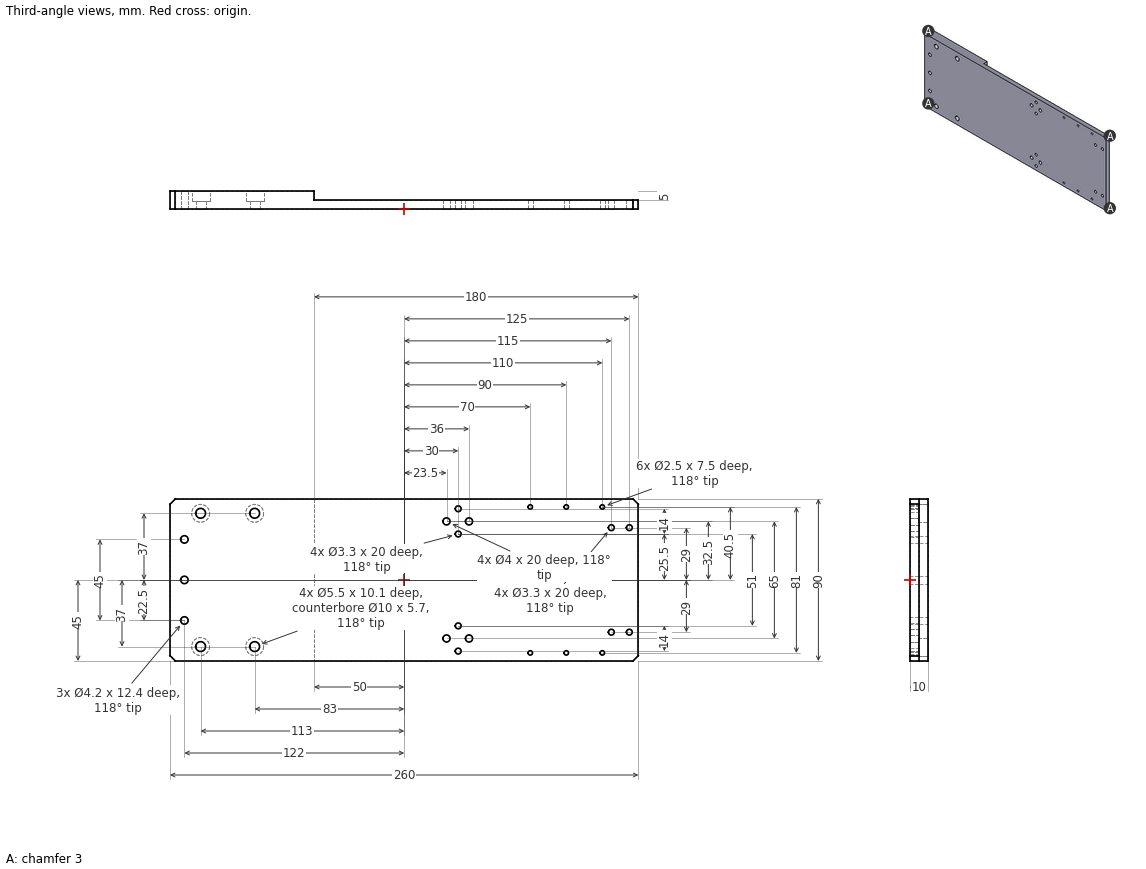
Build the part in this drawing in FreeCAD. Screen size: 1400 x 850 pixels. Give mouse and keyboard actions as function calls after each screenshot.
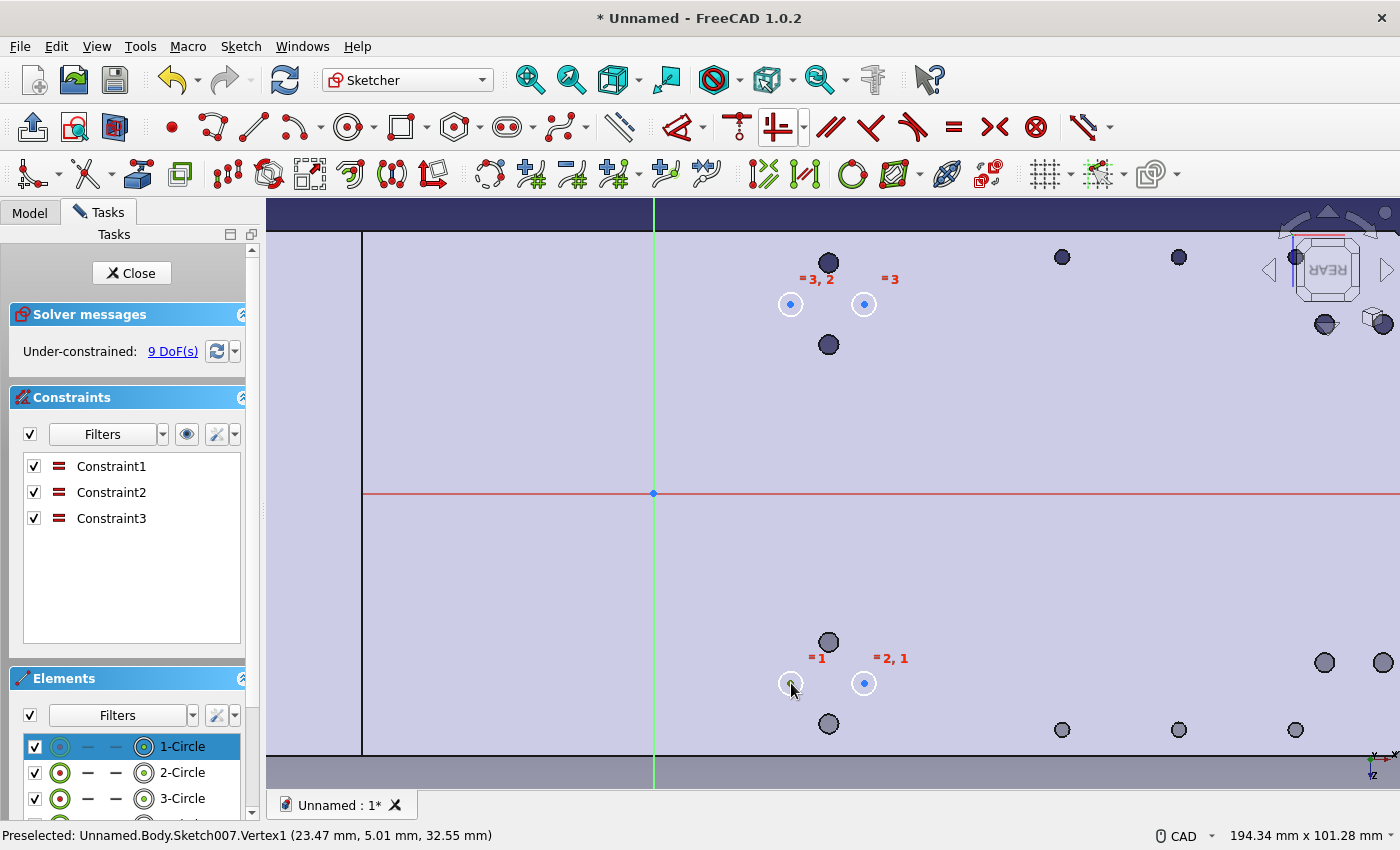
click(864, 683)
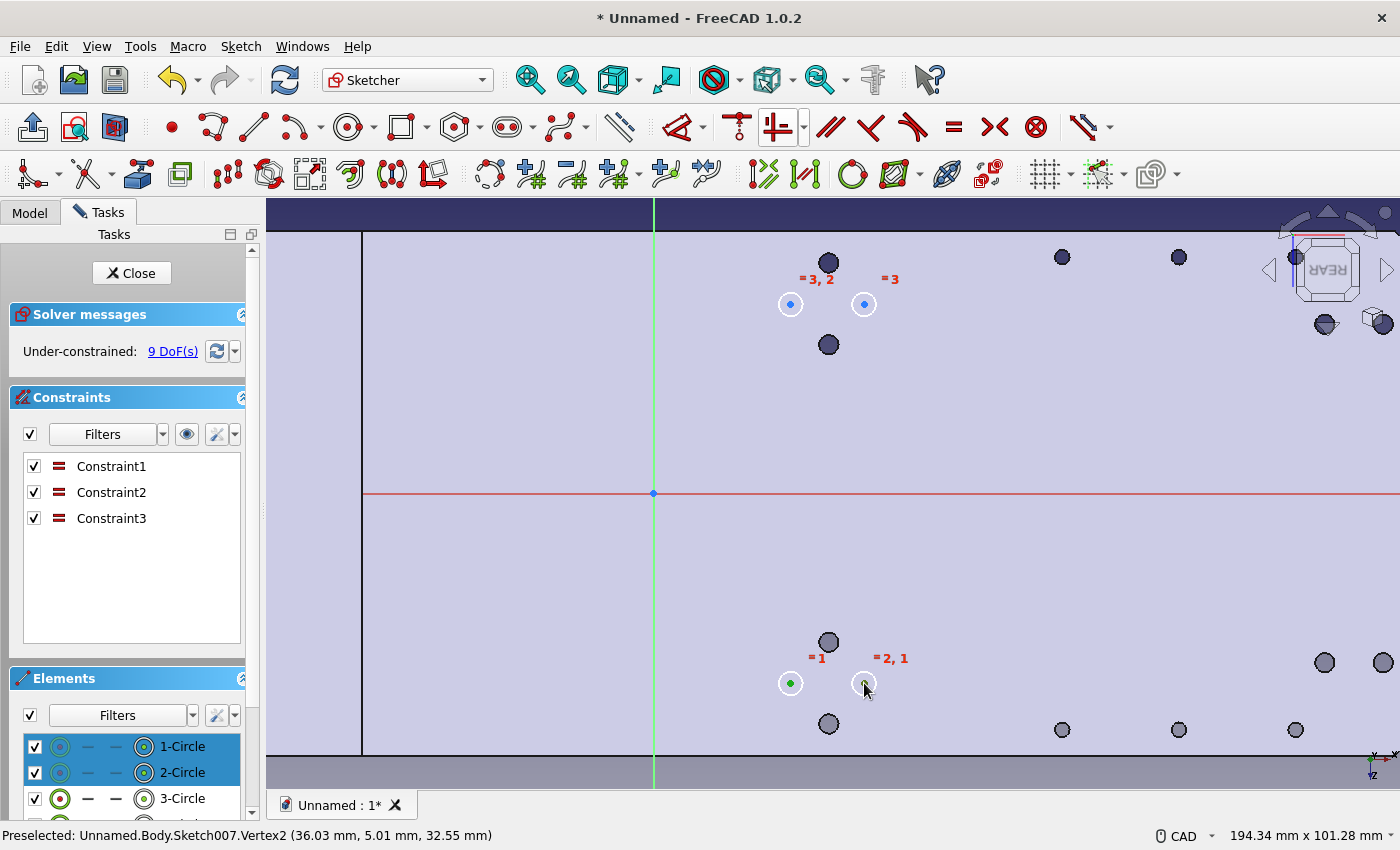
click(804, 128)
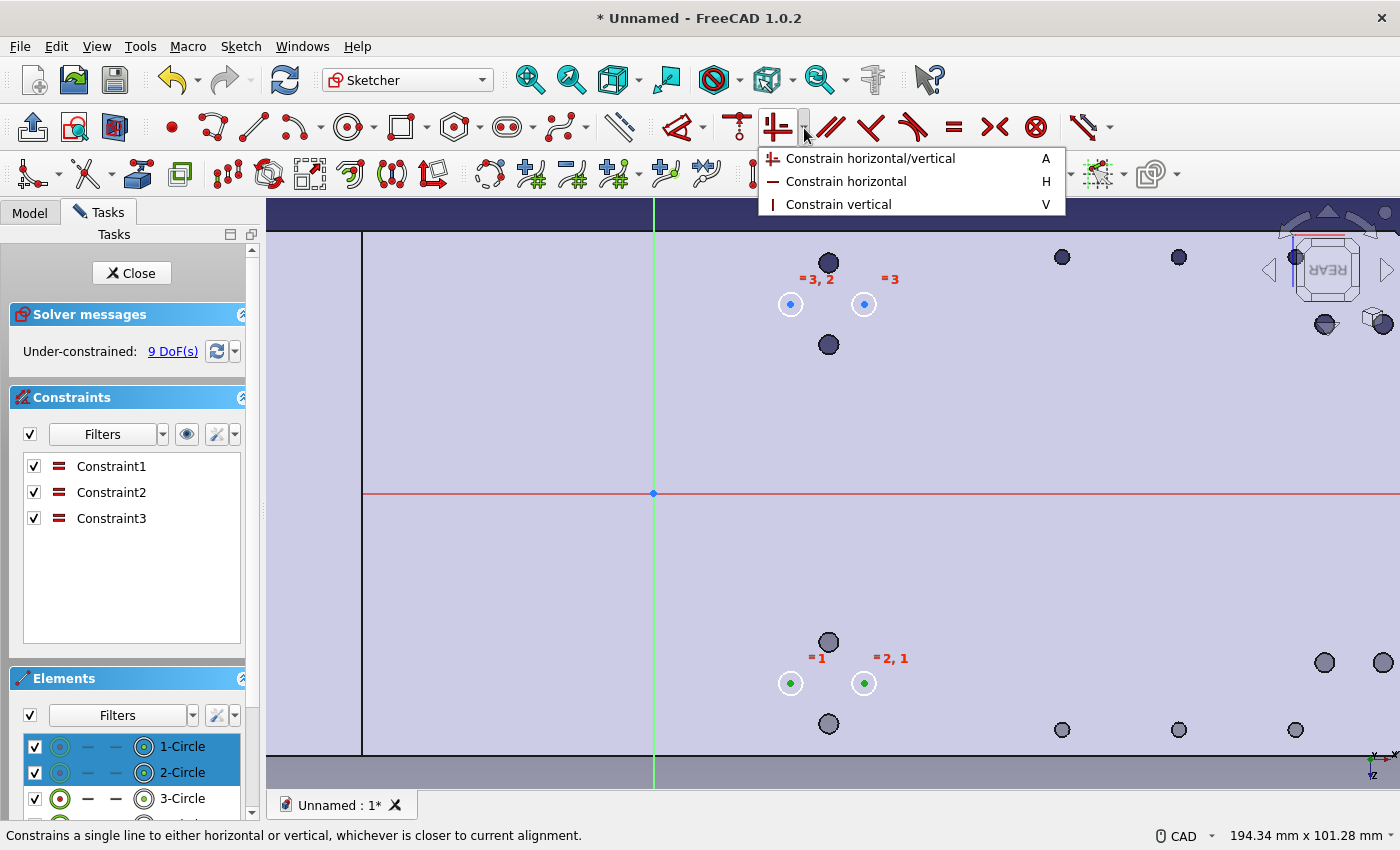
click(912, 182)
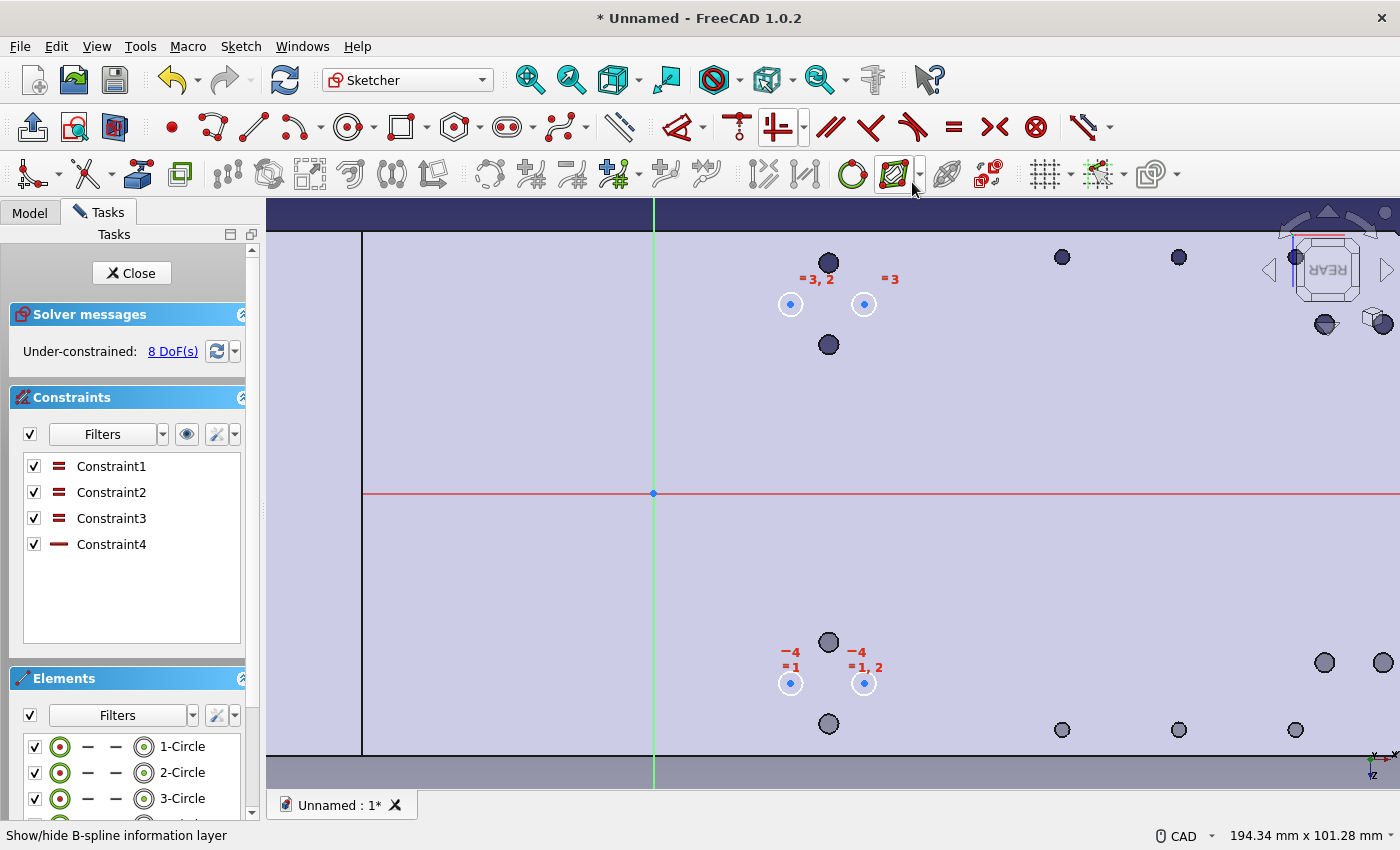
click(791, 683)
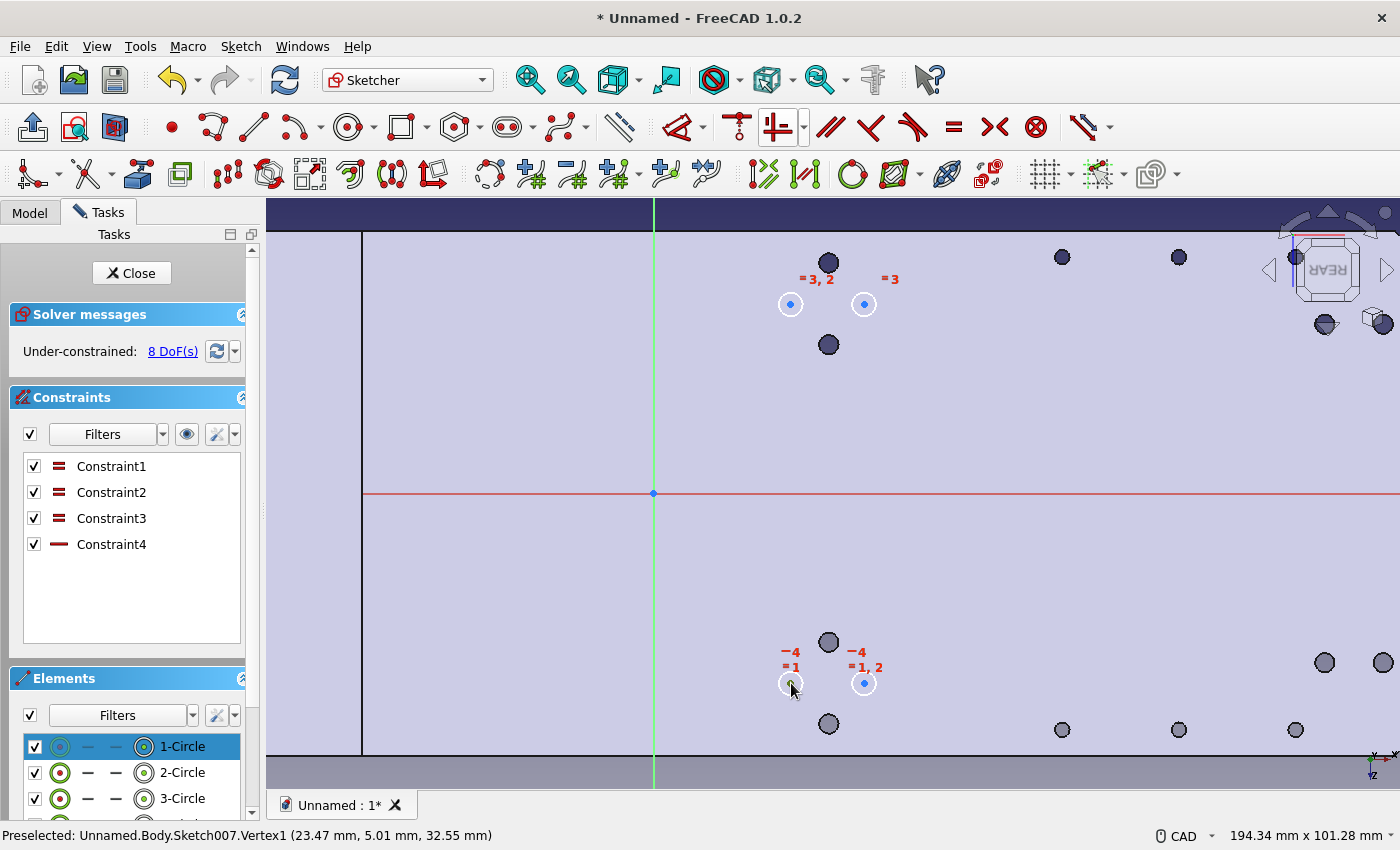
click(791, 304)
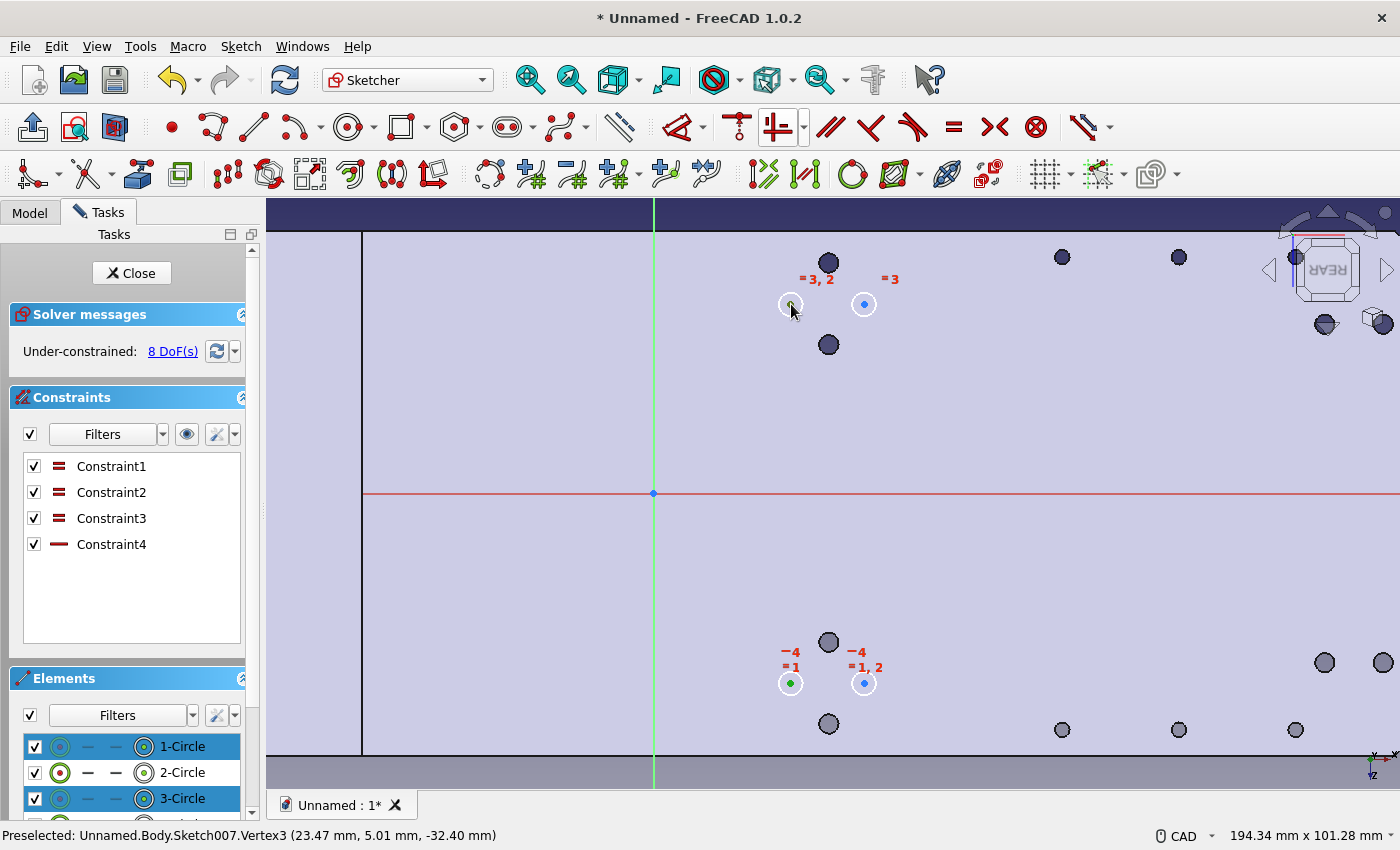
click(804, 128)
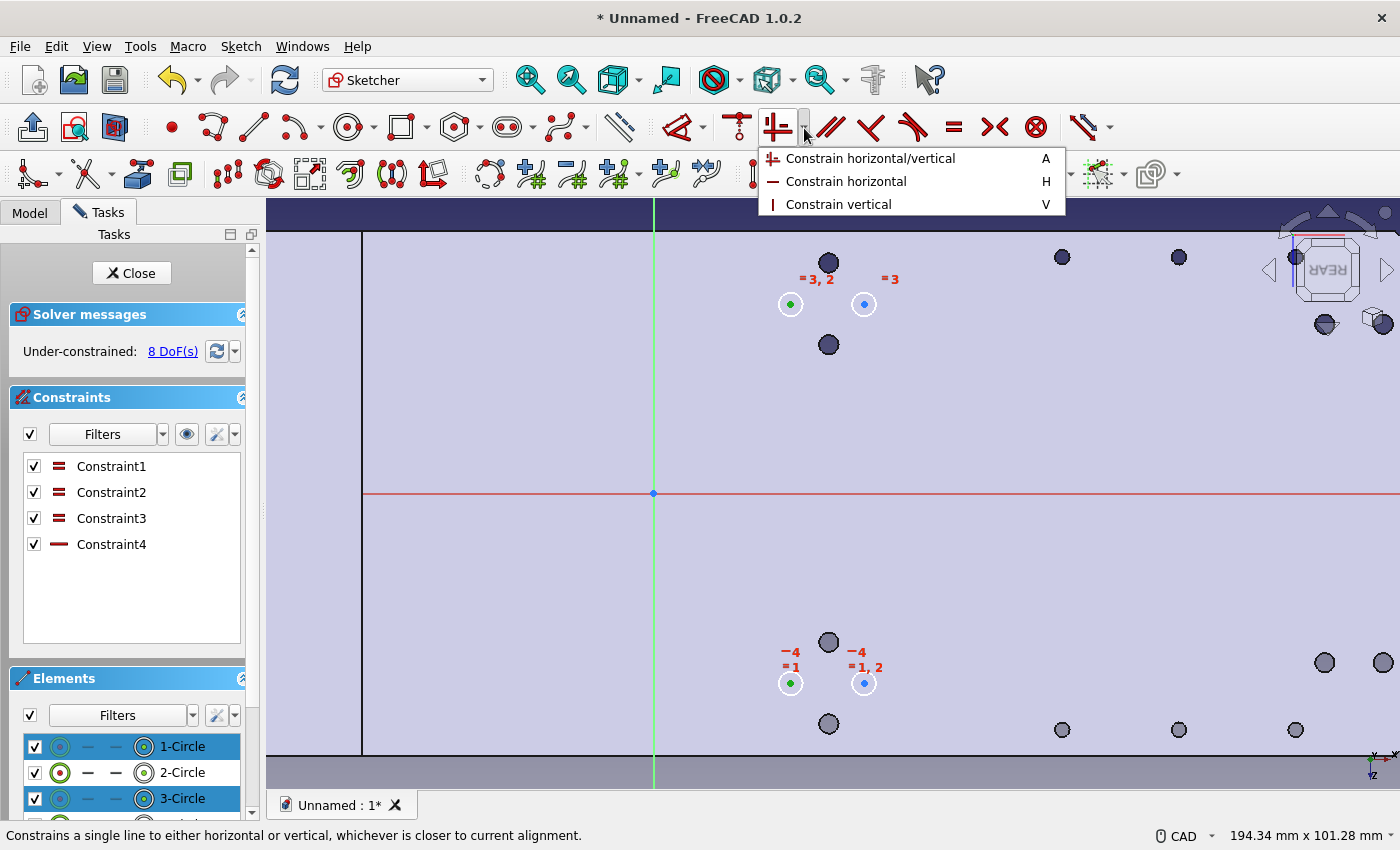
click(912, 204)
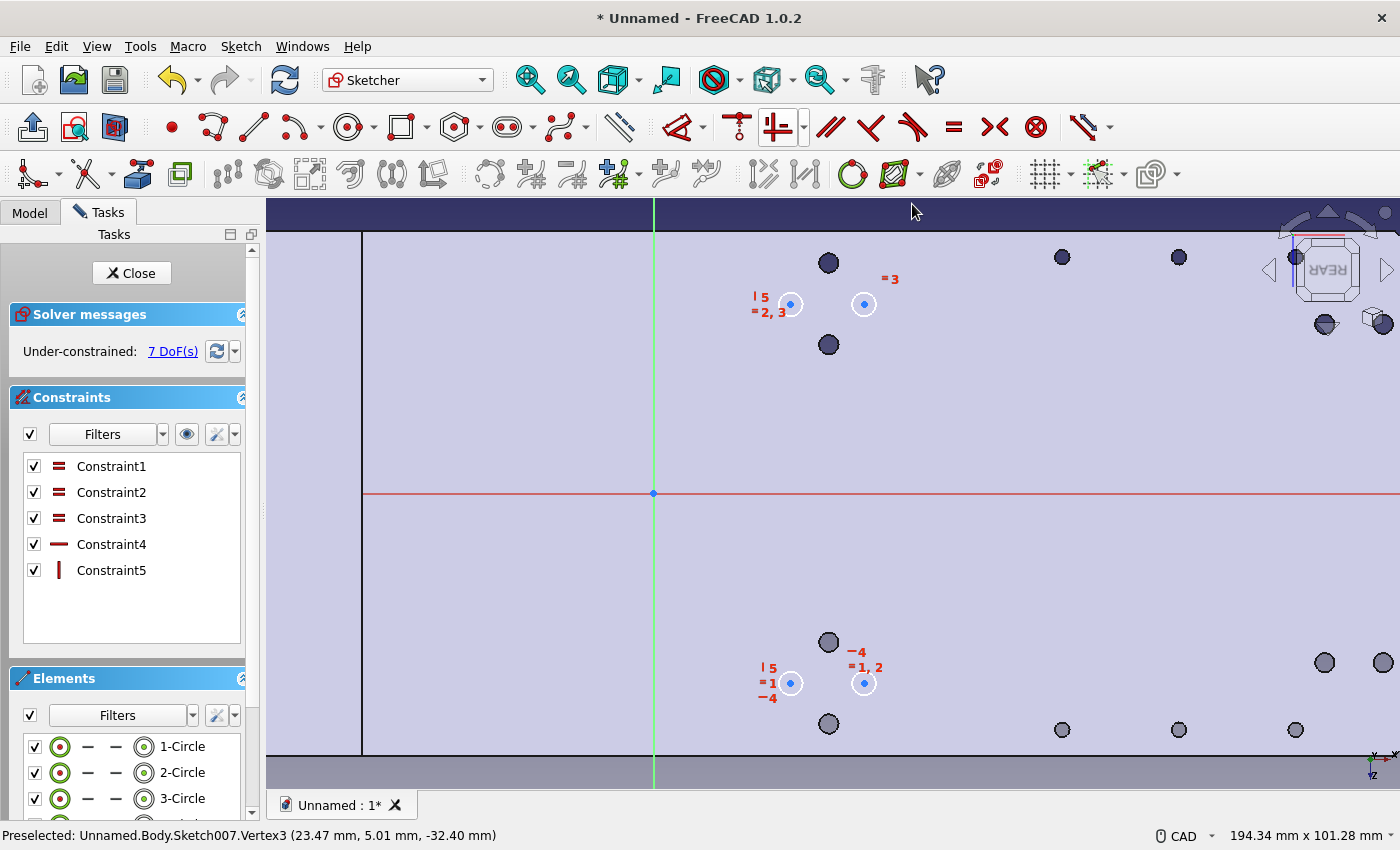
click(864, 683)